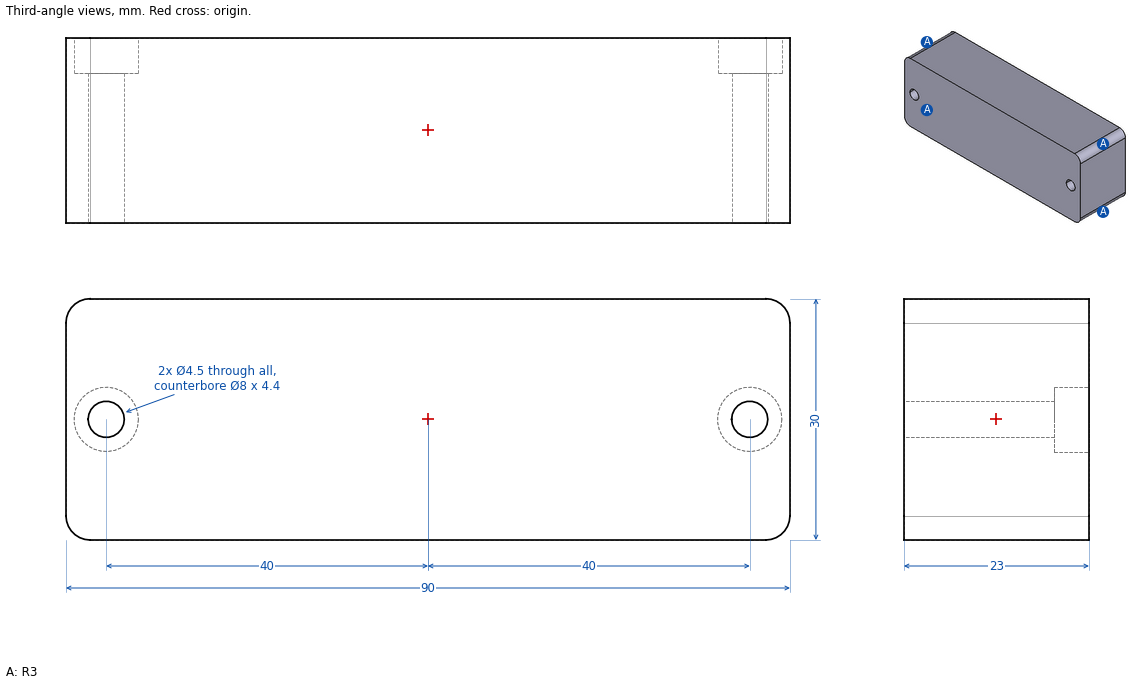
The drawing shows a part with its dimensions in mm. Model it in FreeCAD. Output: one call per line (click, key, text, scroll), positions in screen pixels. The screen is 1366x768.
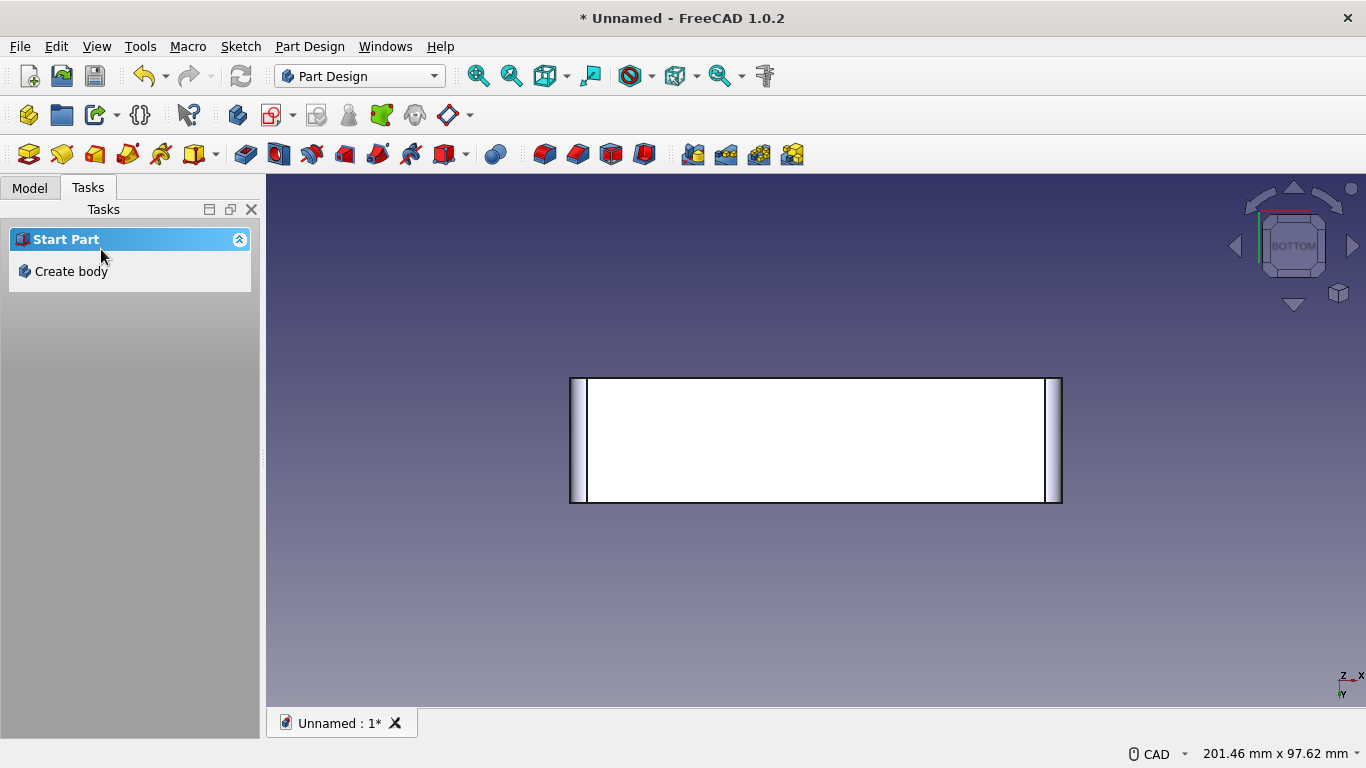
key(0)